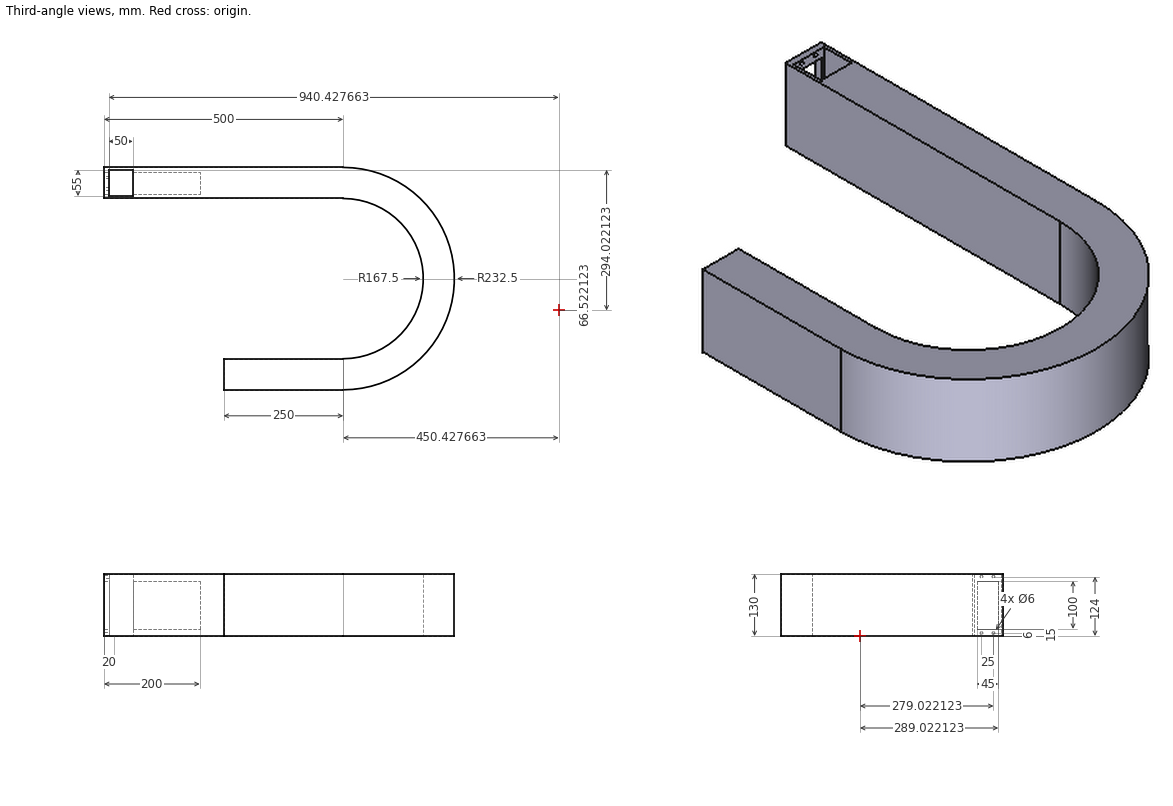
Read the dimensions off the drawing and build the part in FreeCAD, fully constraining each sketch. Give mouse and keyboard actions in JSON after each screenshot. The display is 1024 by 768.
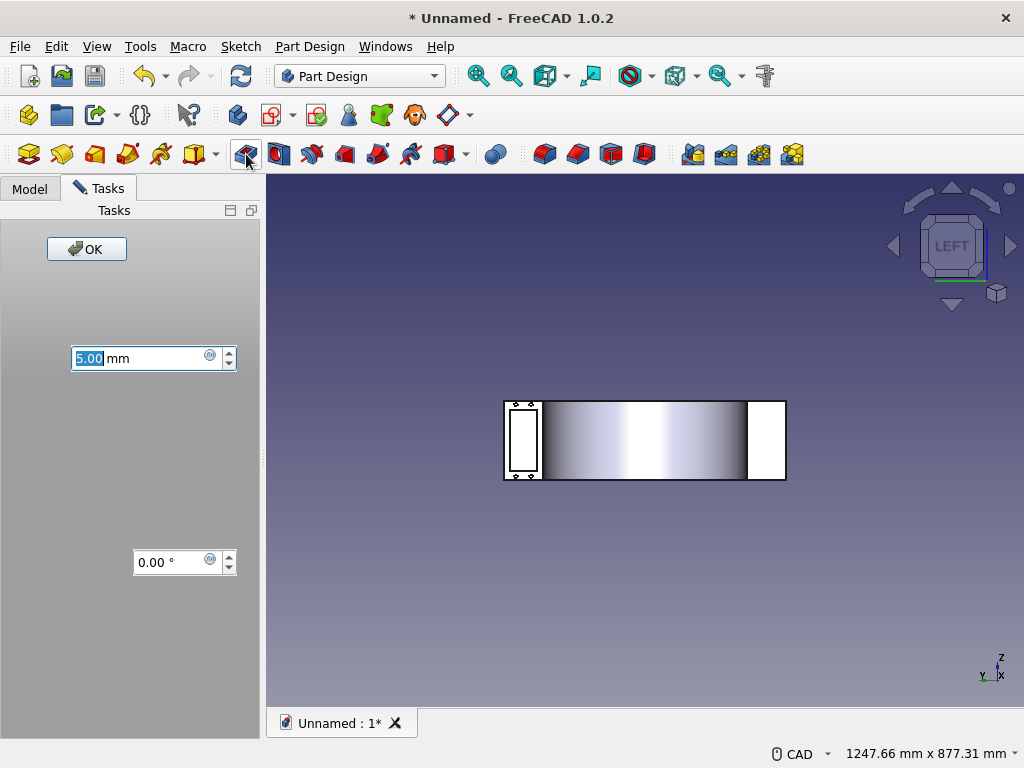
{"action": "type", "text": "200"}
{"action": "key", "text": "Tab"}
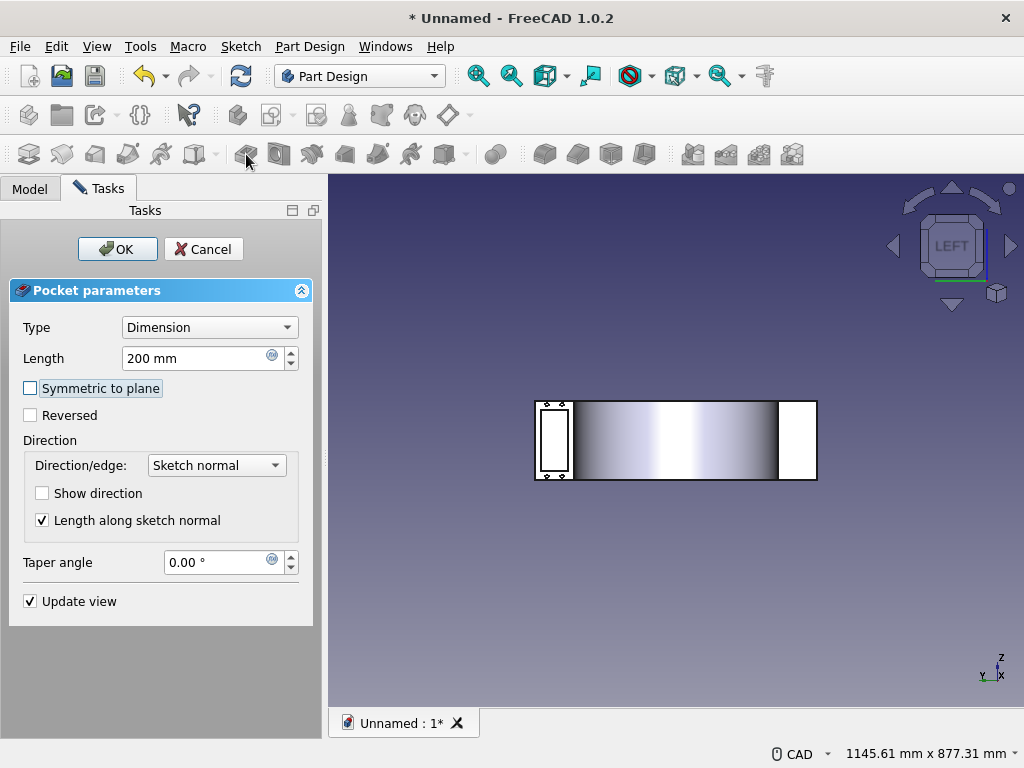
{"action": "left_click", "coordinate": [118, 249]}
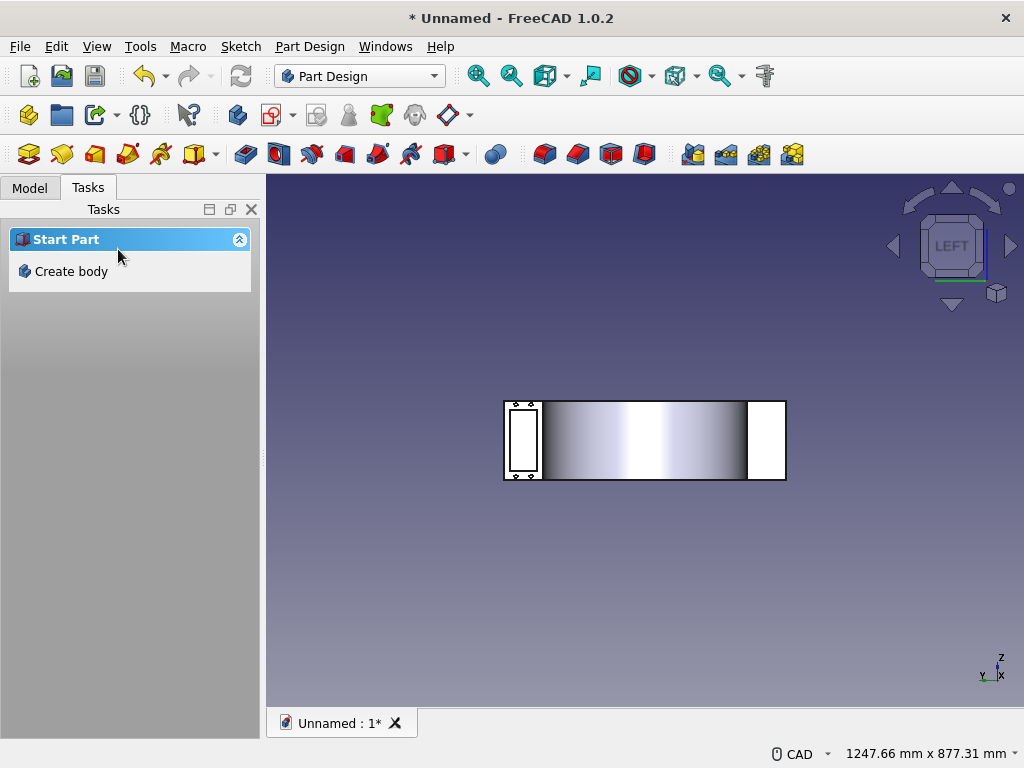
{"action": "key", "text": "0"}